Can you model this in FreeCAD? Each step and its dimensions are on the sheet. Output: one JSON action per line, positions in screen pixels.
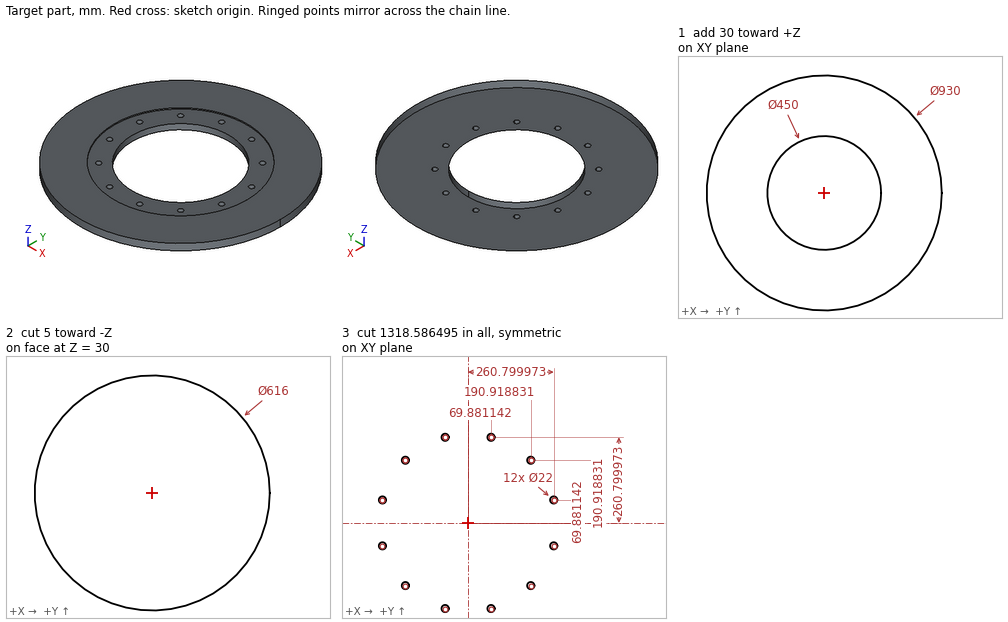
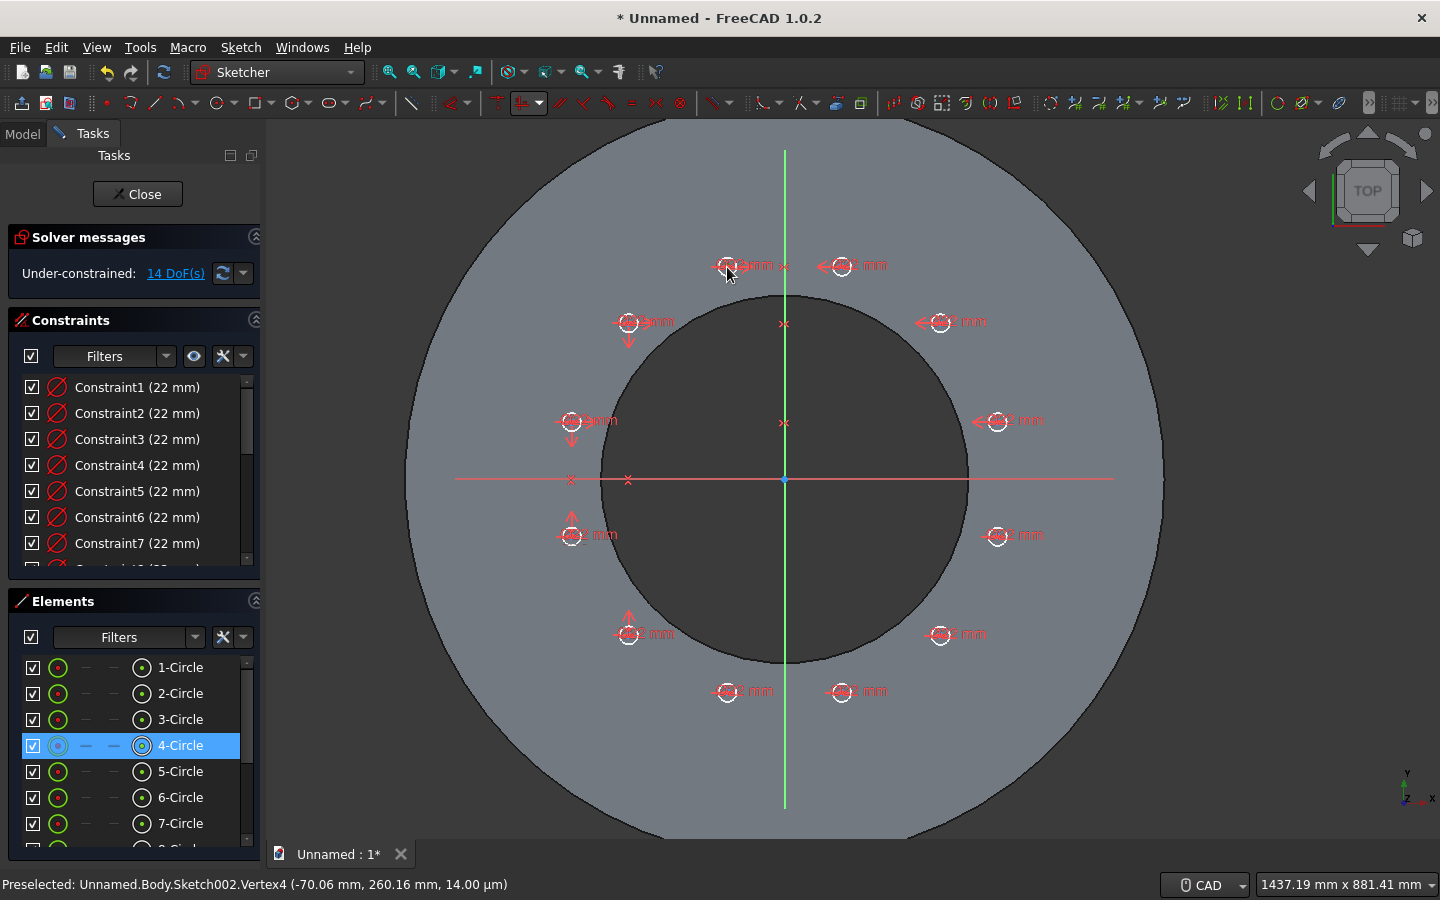
{"action": "left_click", "coordinate": [728, 693]}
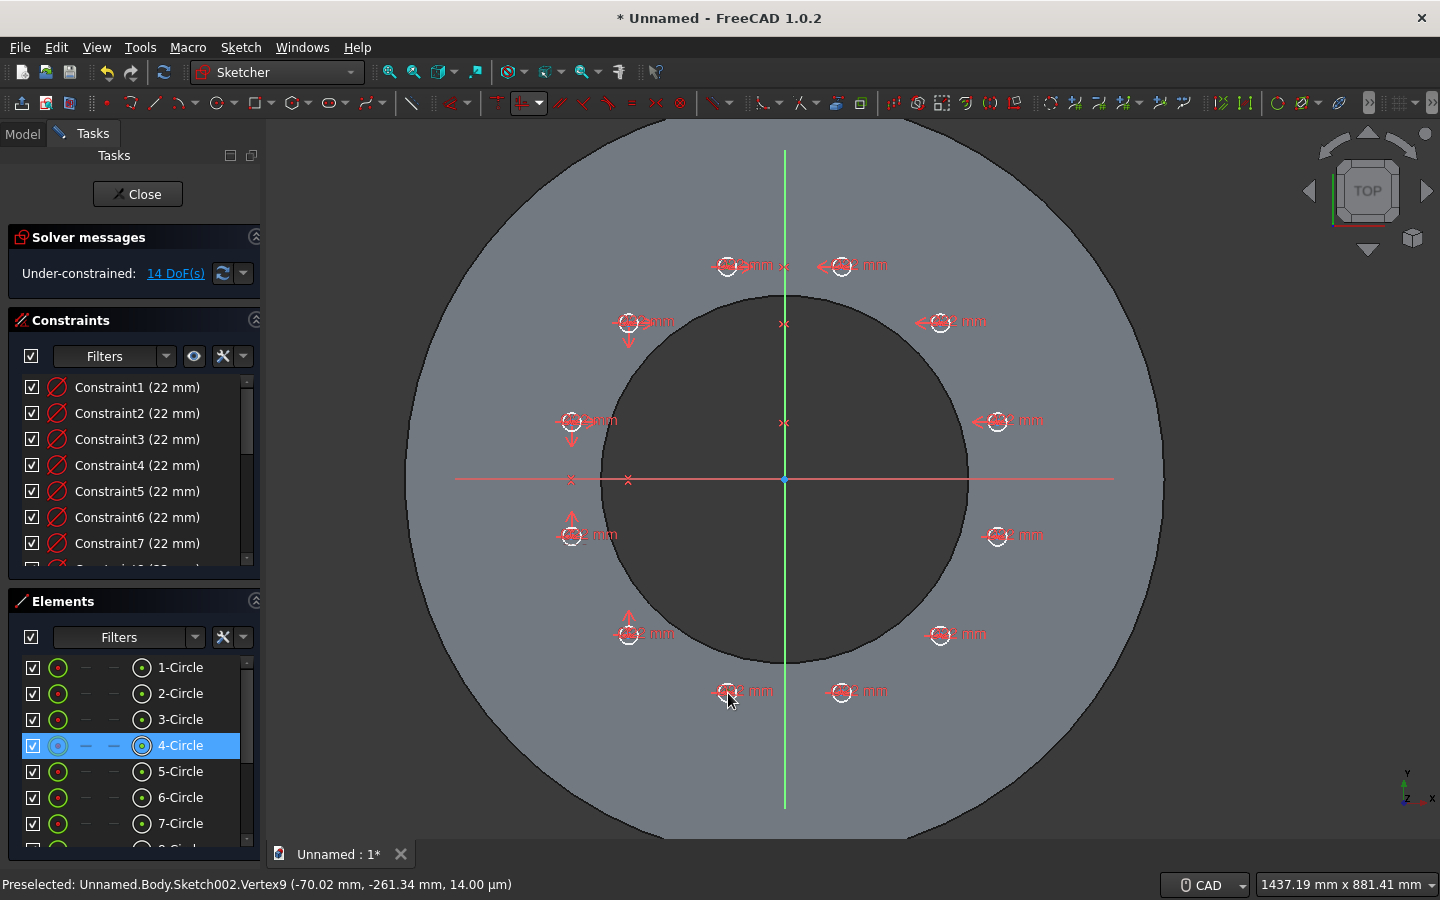
{"action": "left_click", "coordinate": [504, 479]}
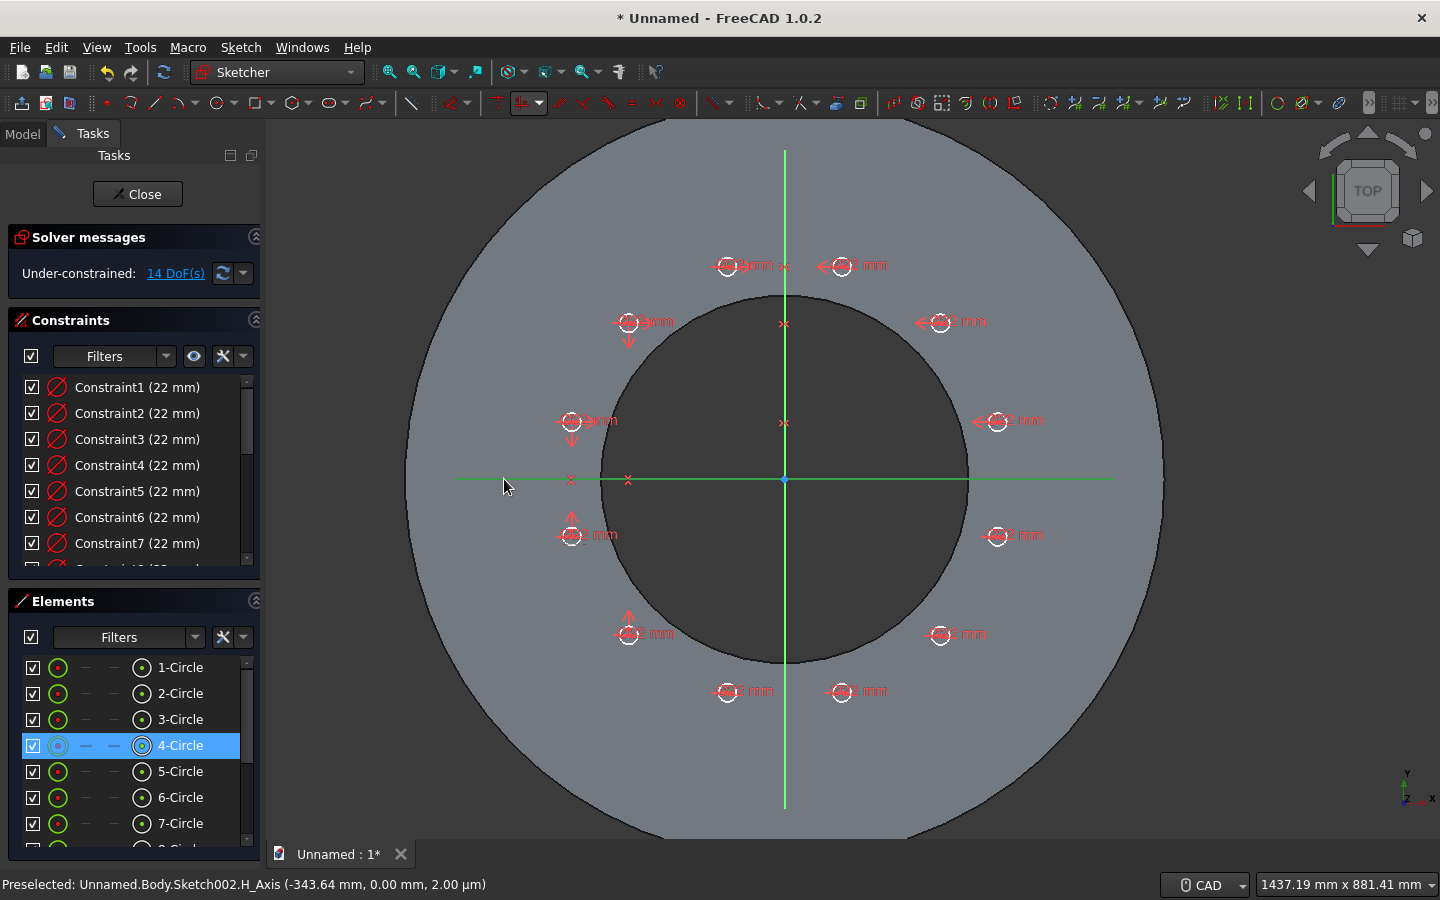
{"action": "left_click", "coordinate": [656, 104]}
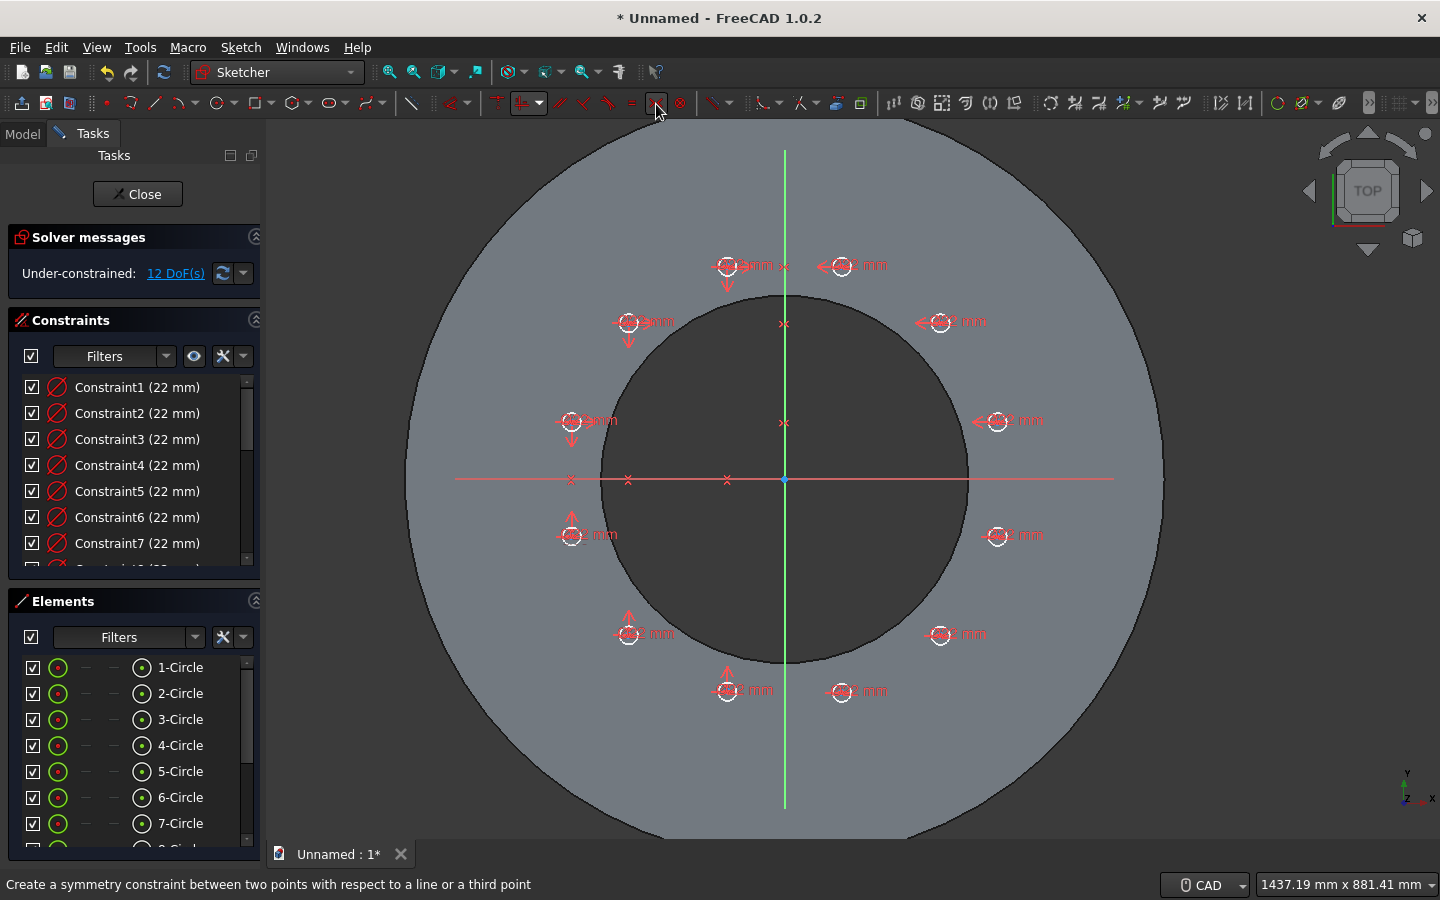
{"action": "left_click", "coordinate": [842, 267]}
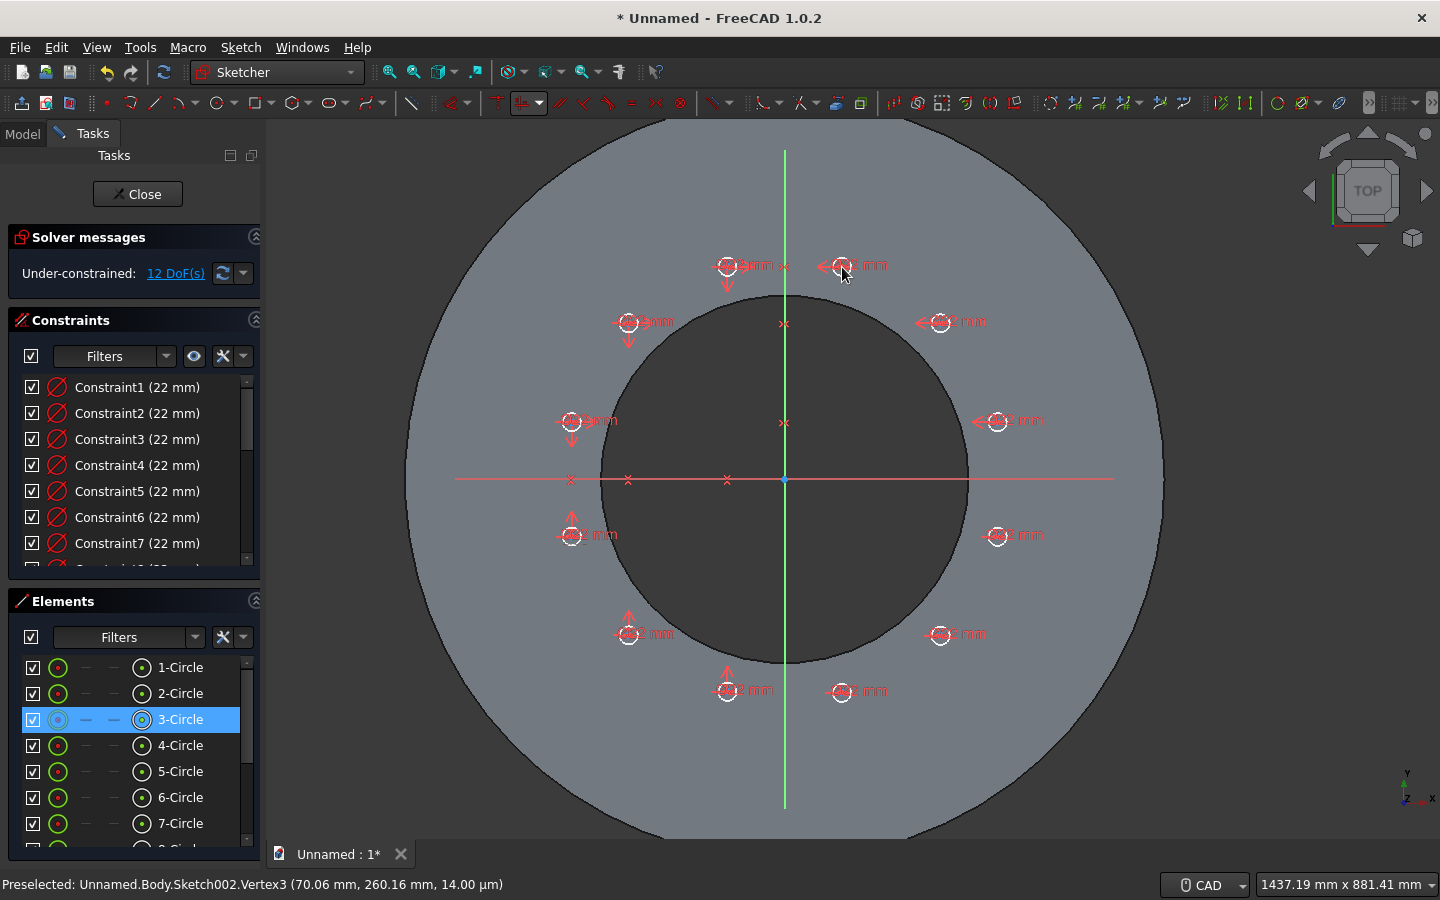
{"action": "left_click", "coordinate": [842, 693]}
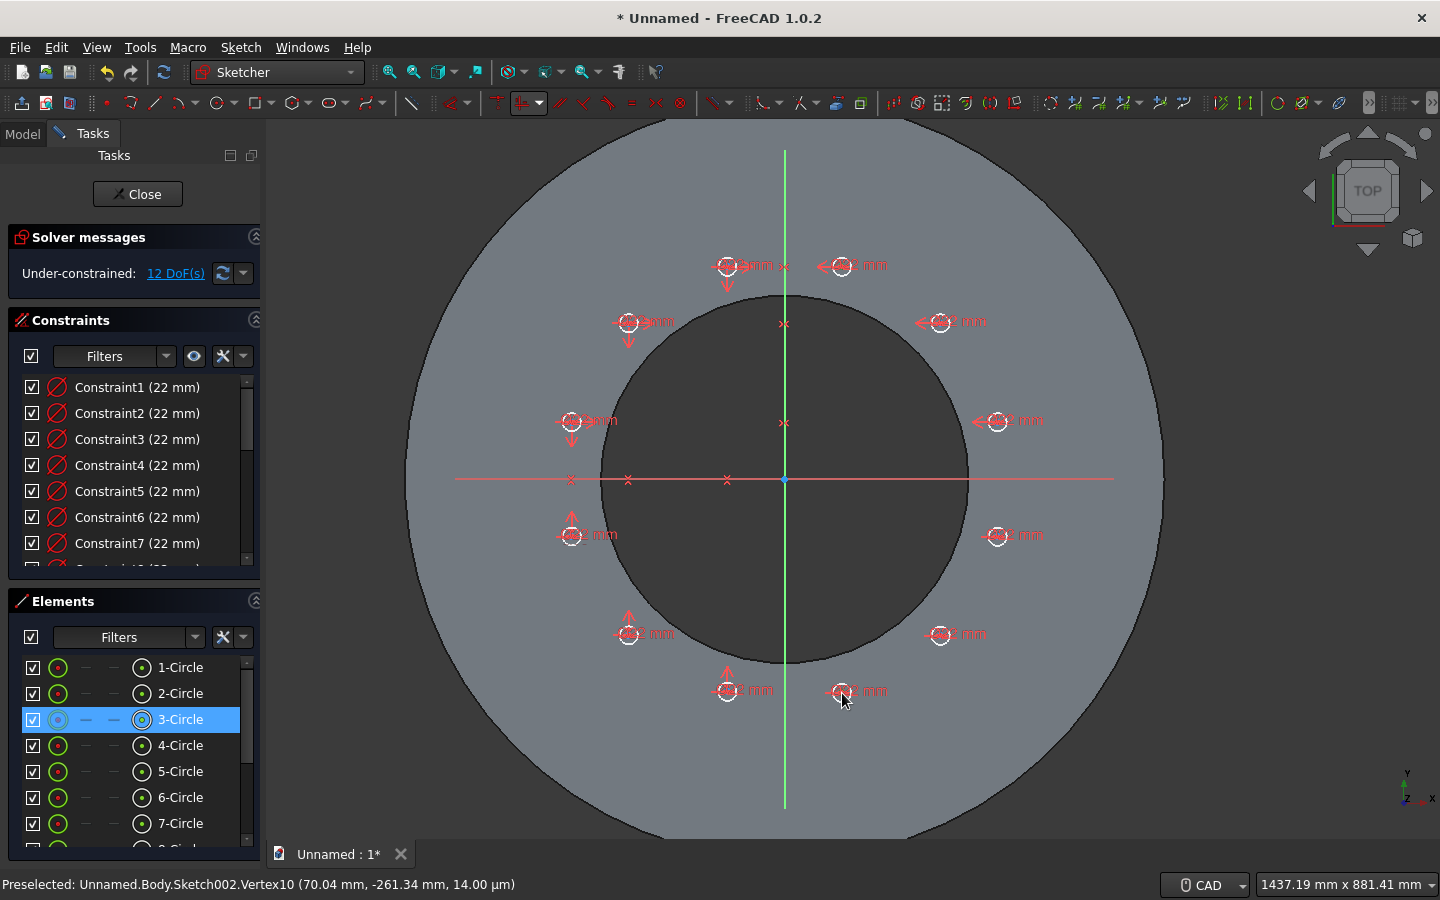
{"action": "left_click", "coordinate": [504, 479]}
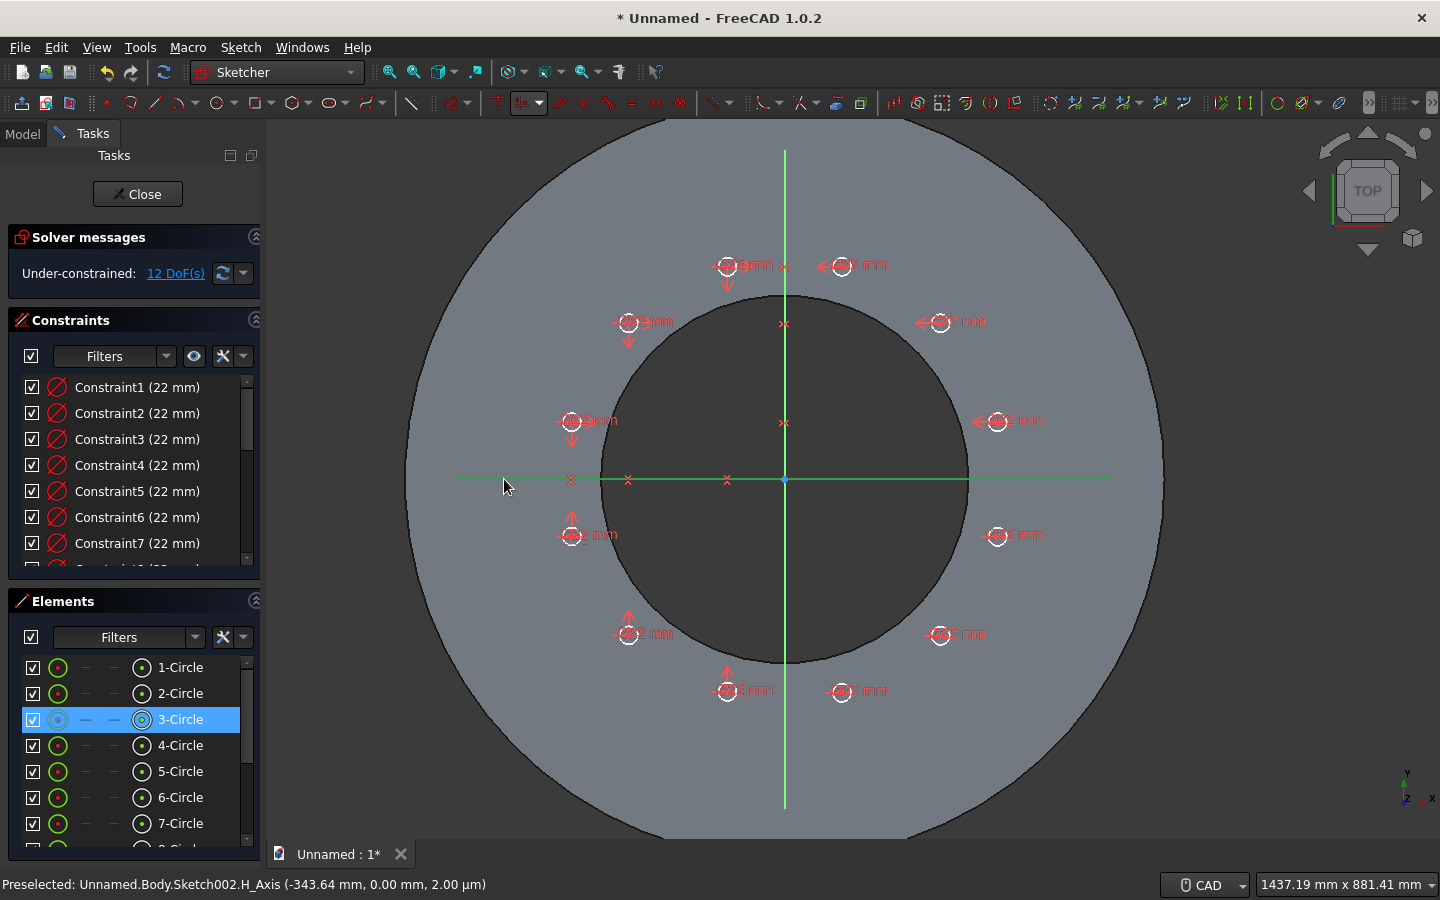
{"action": "left_click", "coordinate": [656, 104]}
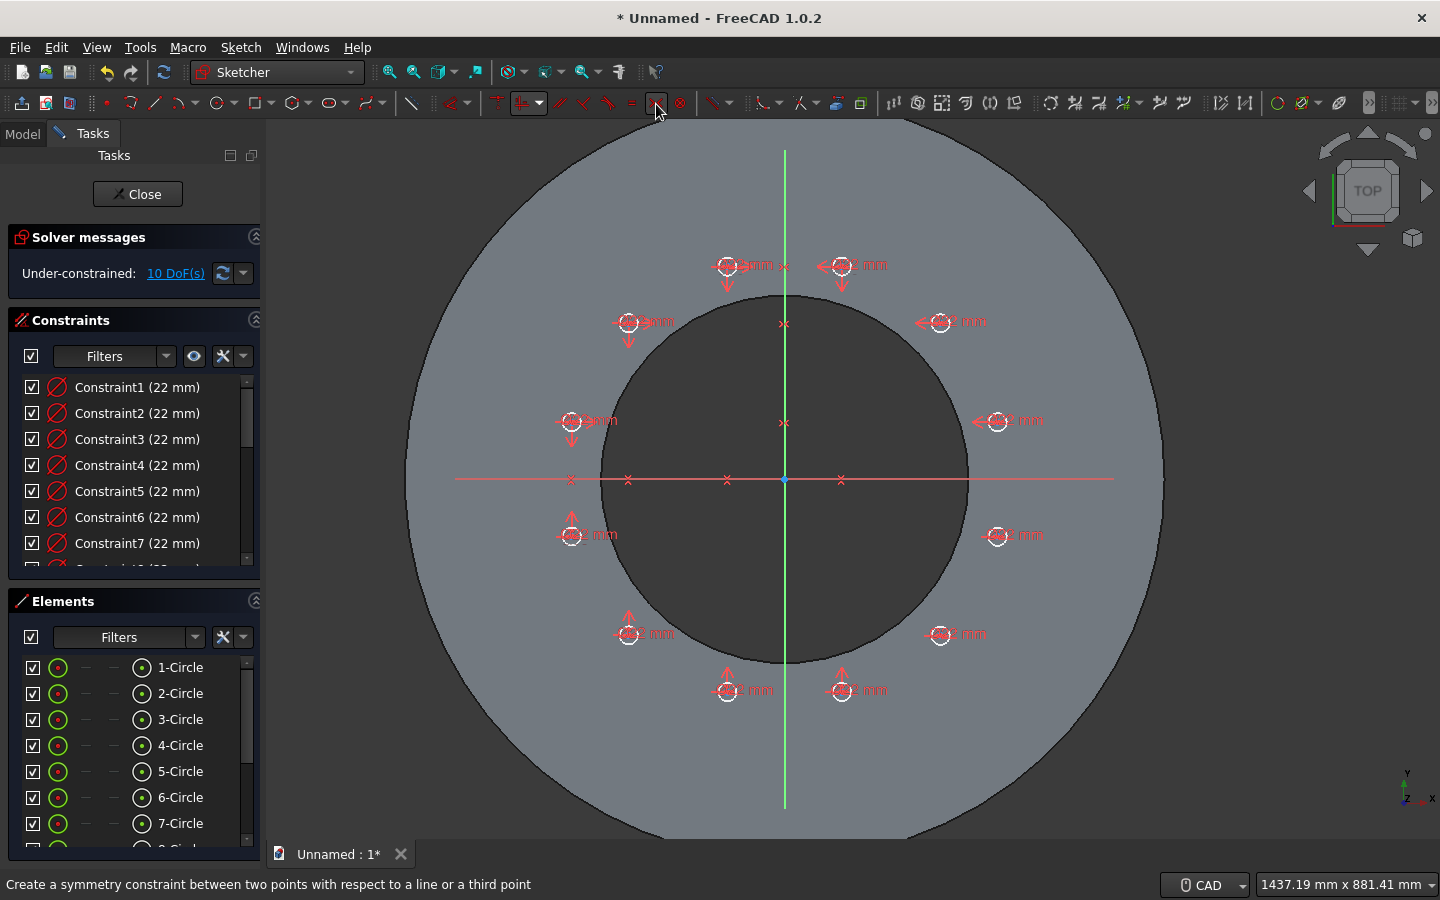
{"action": "left_click", "coordinate": [941, 323]}